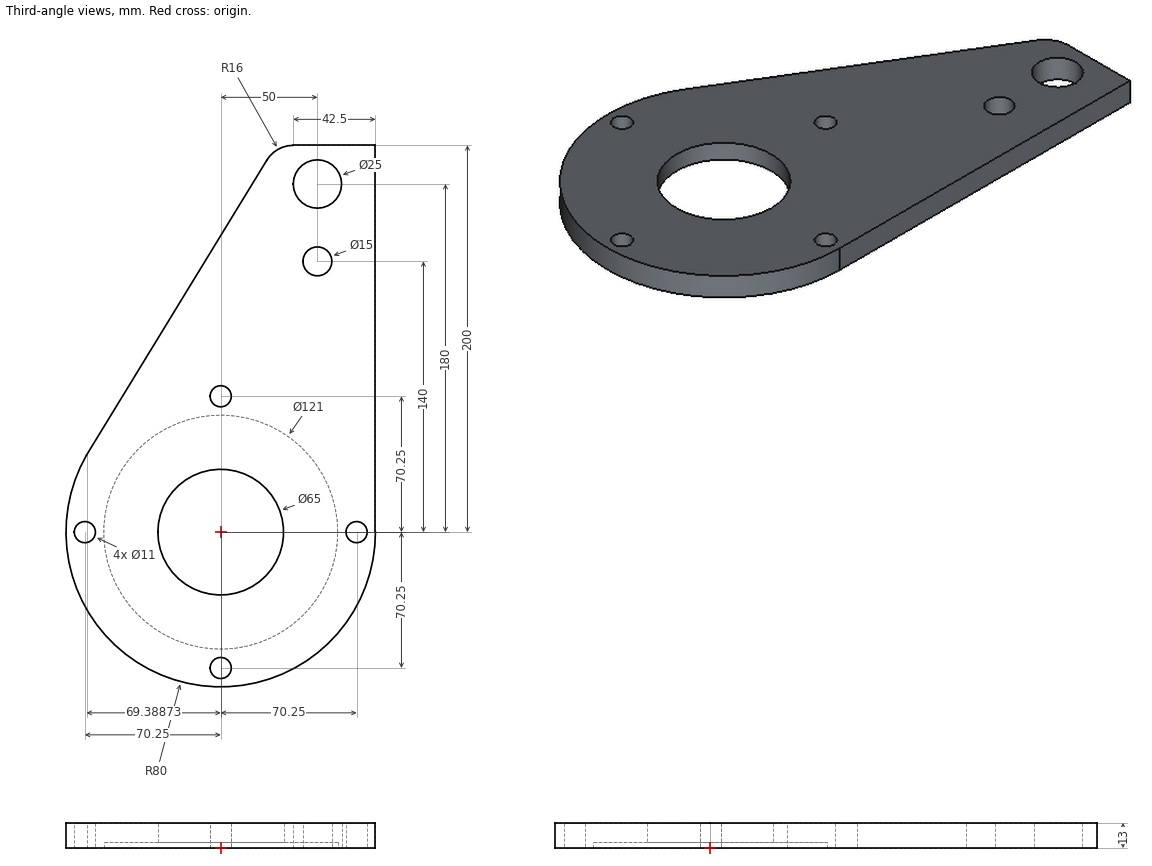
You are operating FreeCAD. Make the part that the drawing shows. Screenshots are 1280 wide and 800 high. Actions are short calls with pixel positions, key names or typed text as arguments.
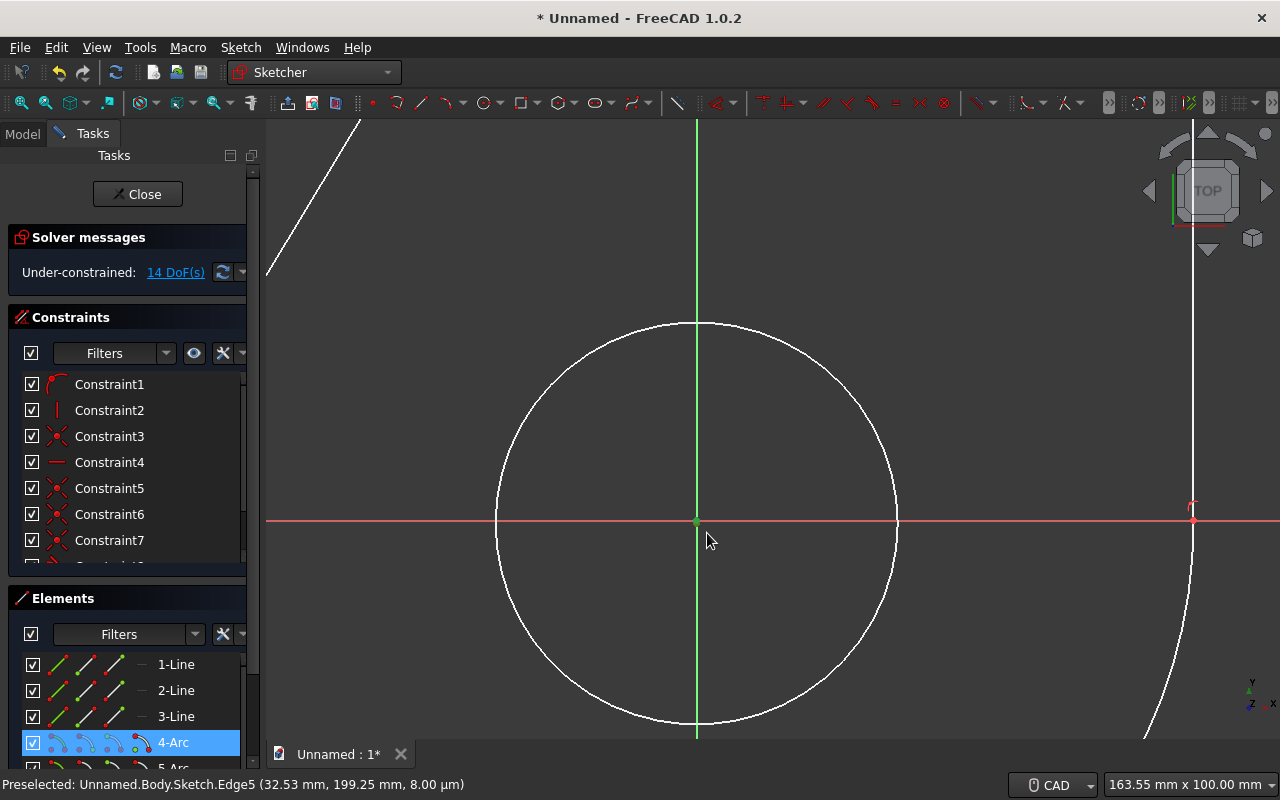
click(764, 104)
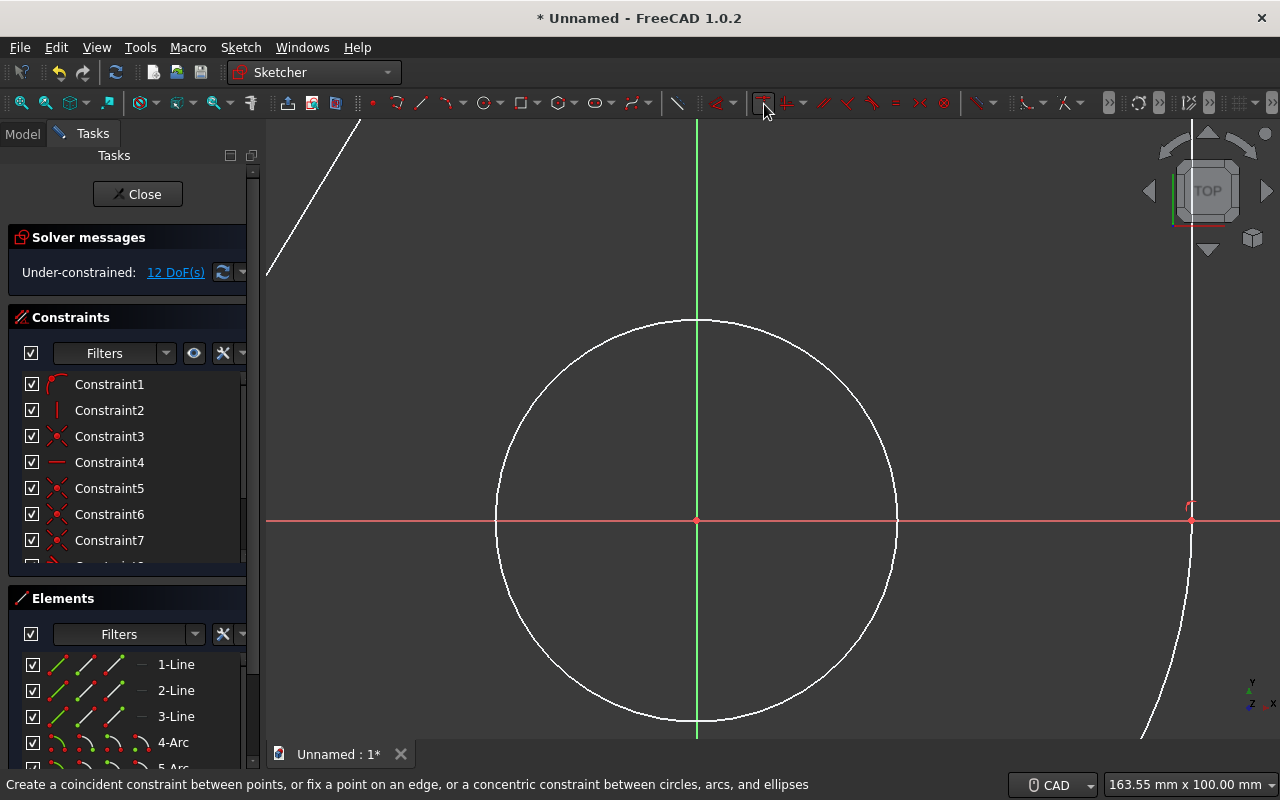
click(716, 104)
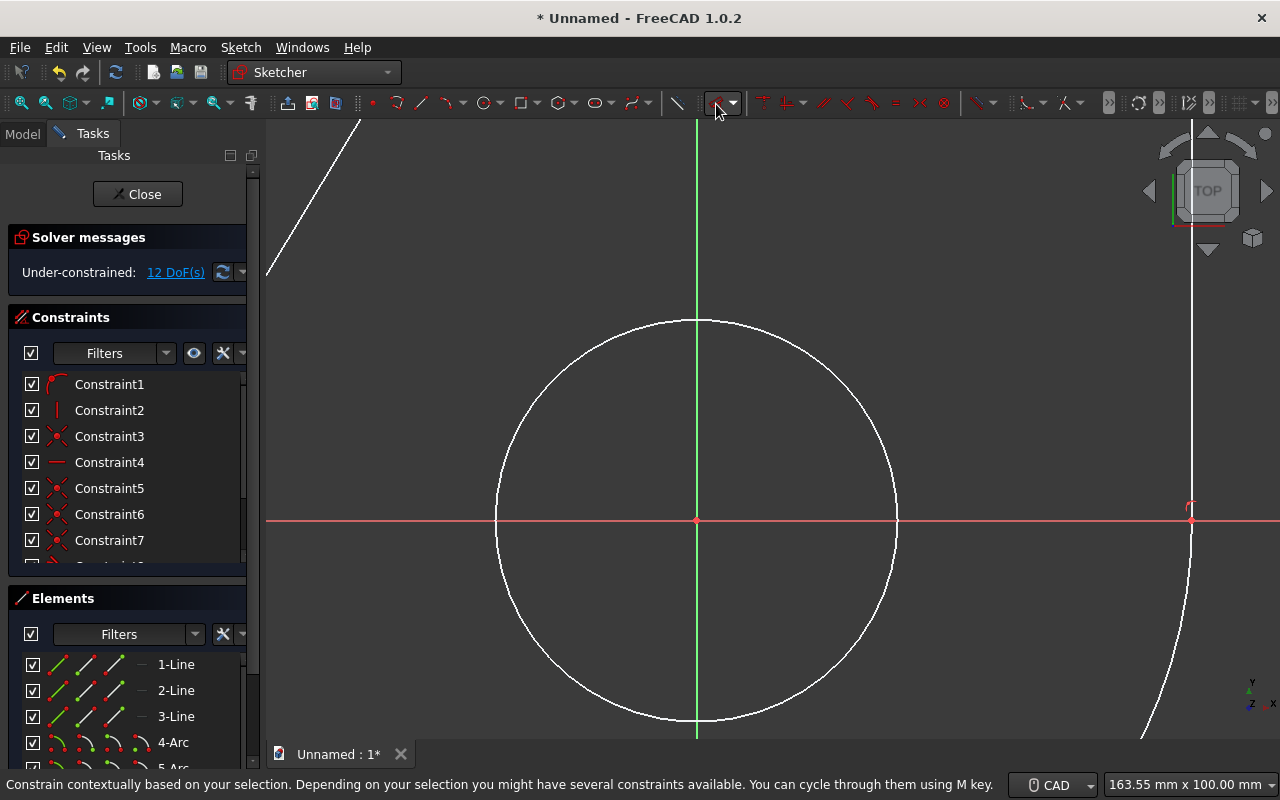
scroll(696, 523, down, 7)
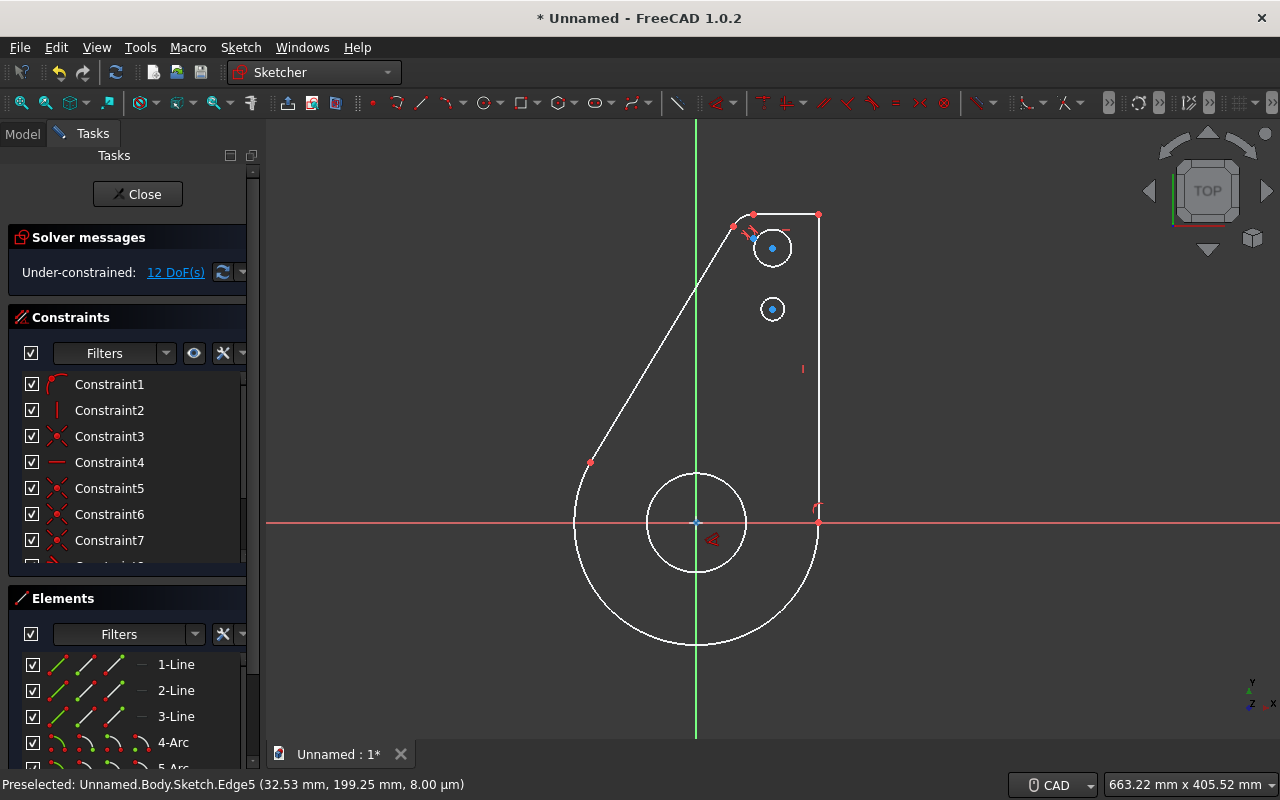
click(594, 590)
click(567, 608)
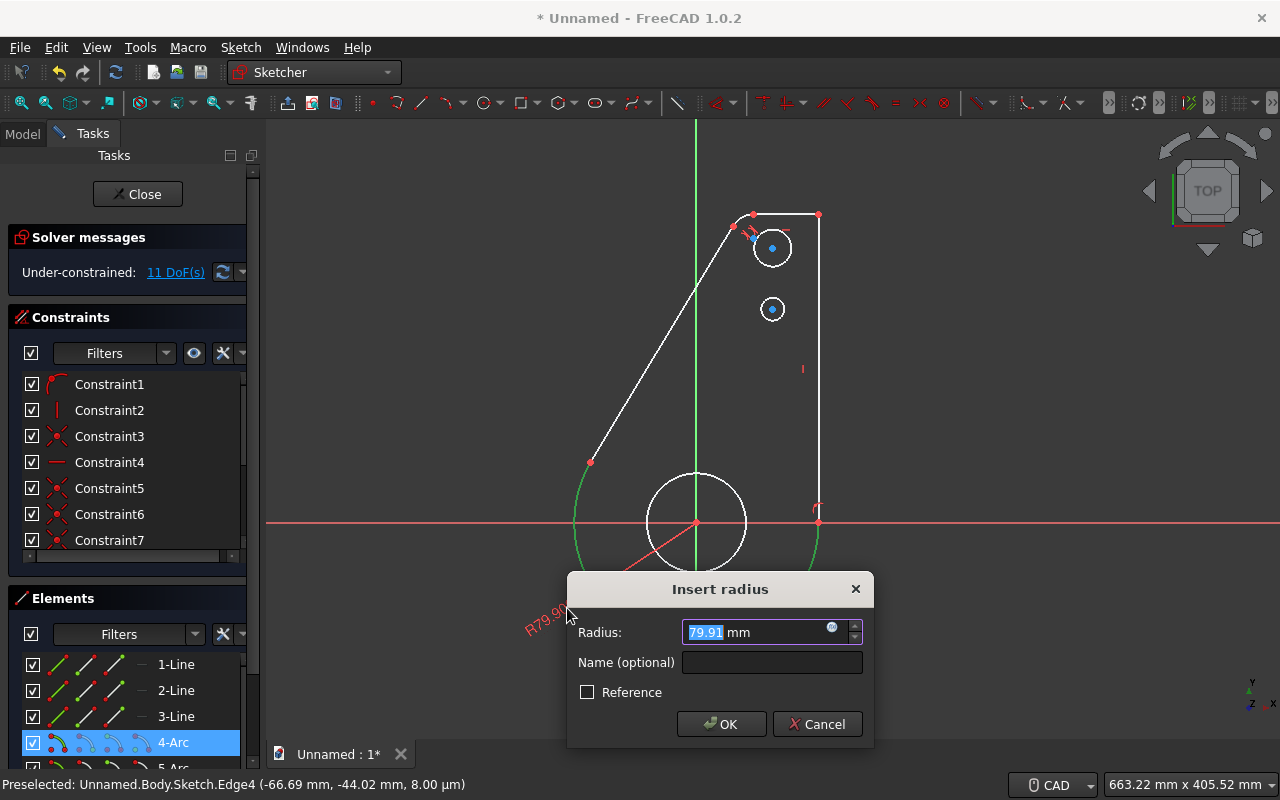
text(80)
key(Return)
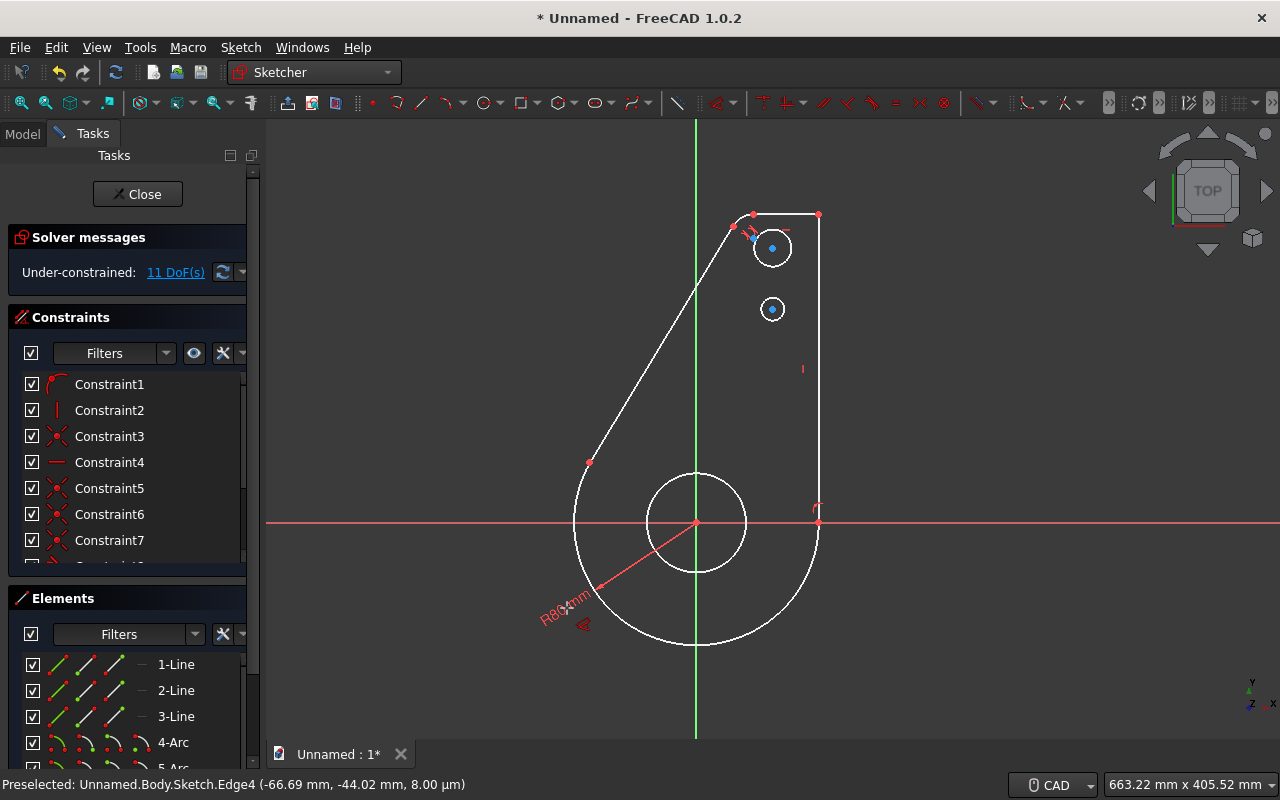
scroll(742, 217, up, 3)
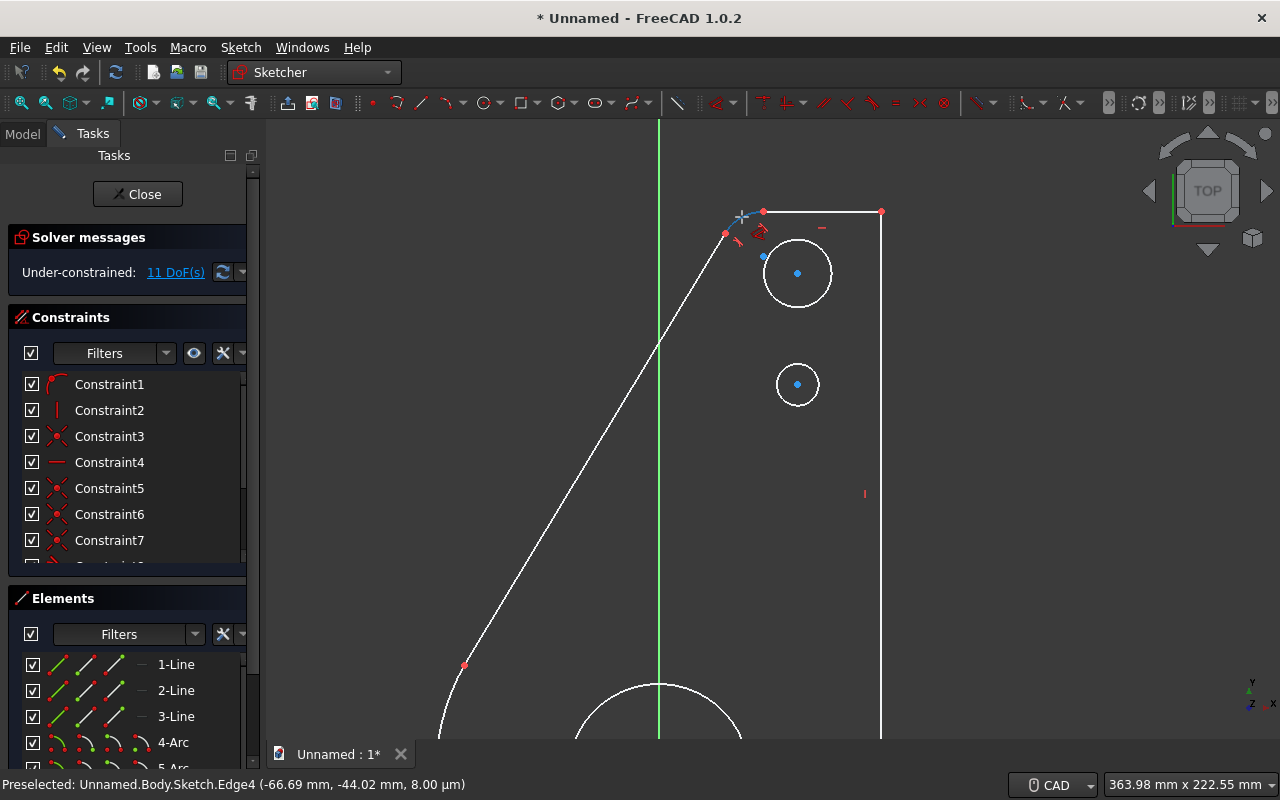
click(742, 218)
click(726, 190)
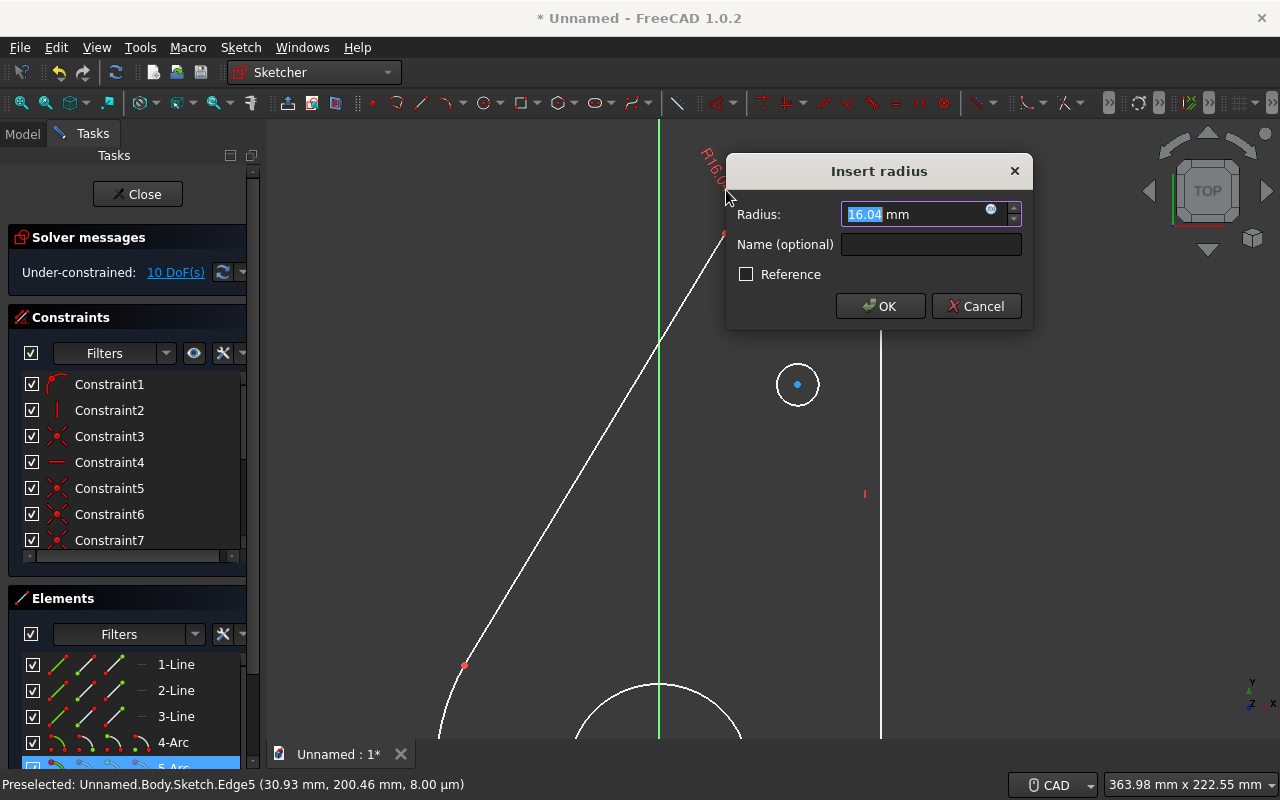
text(16)
key(Return)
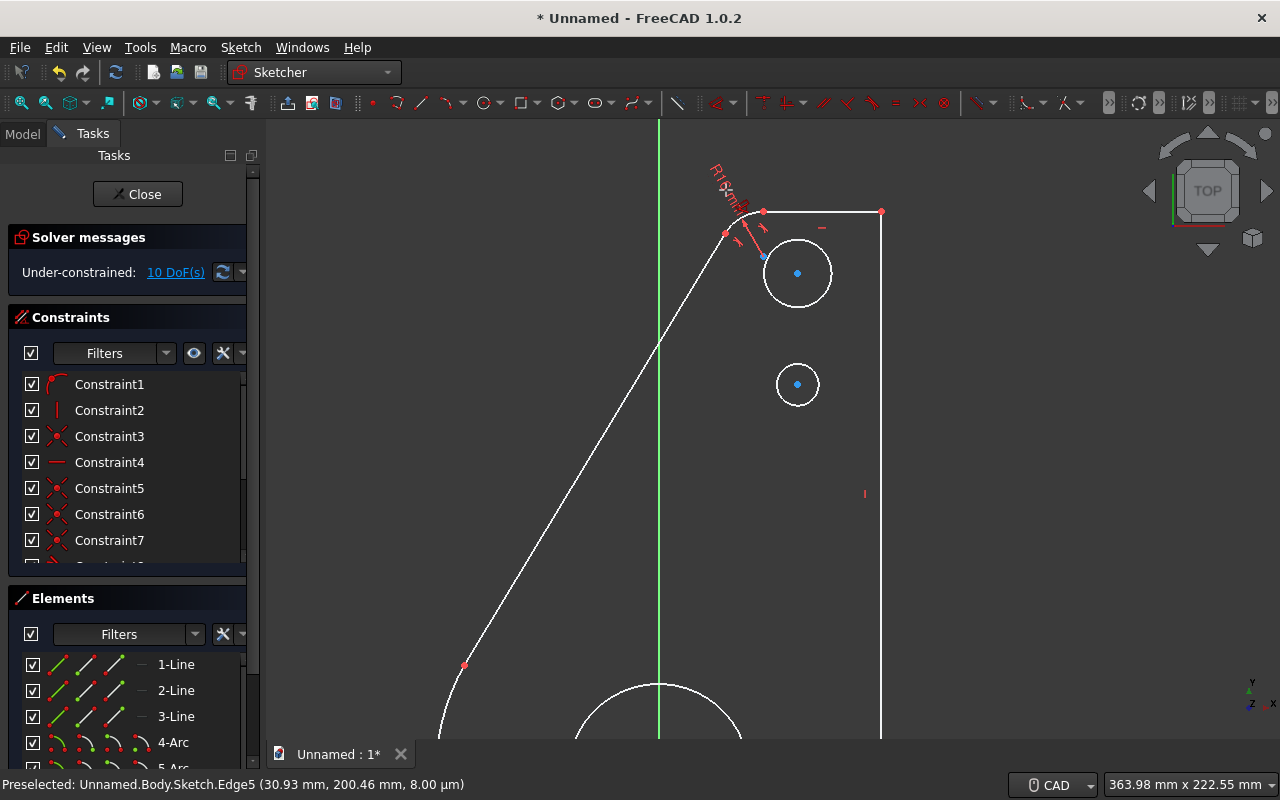
click(722, 710)
click(744, 687)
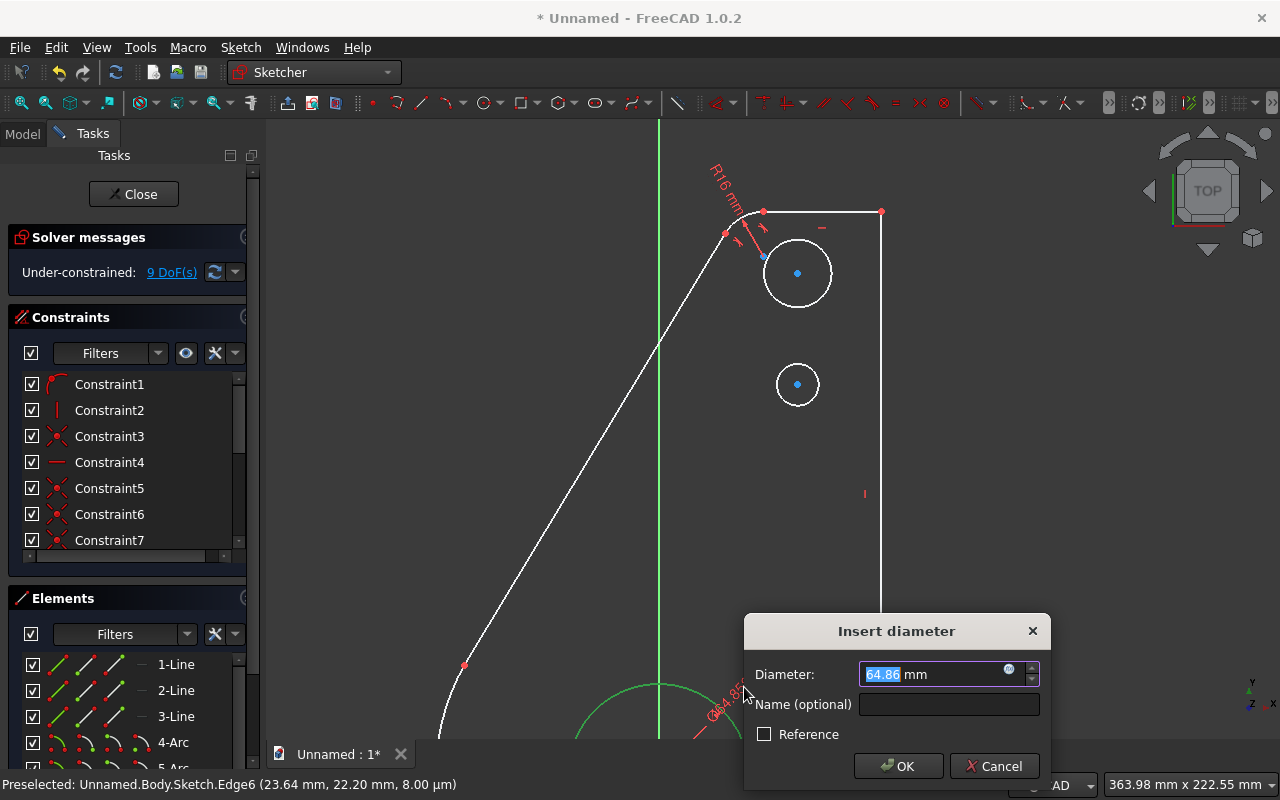
text(65)
key(Return)